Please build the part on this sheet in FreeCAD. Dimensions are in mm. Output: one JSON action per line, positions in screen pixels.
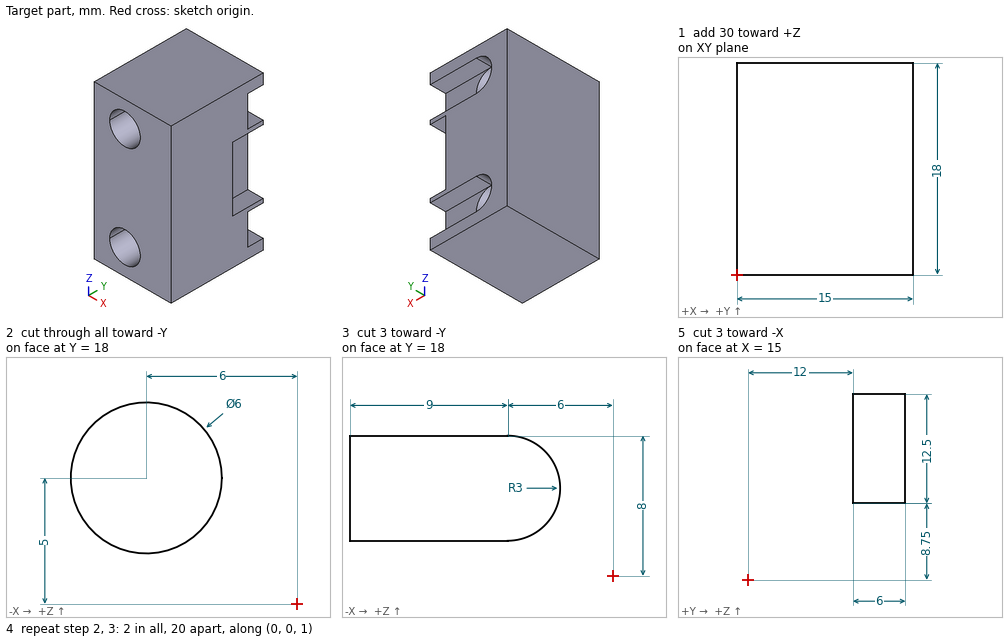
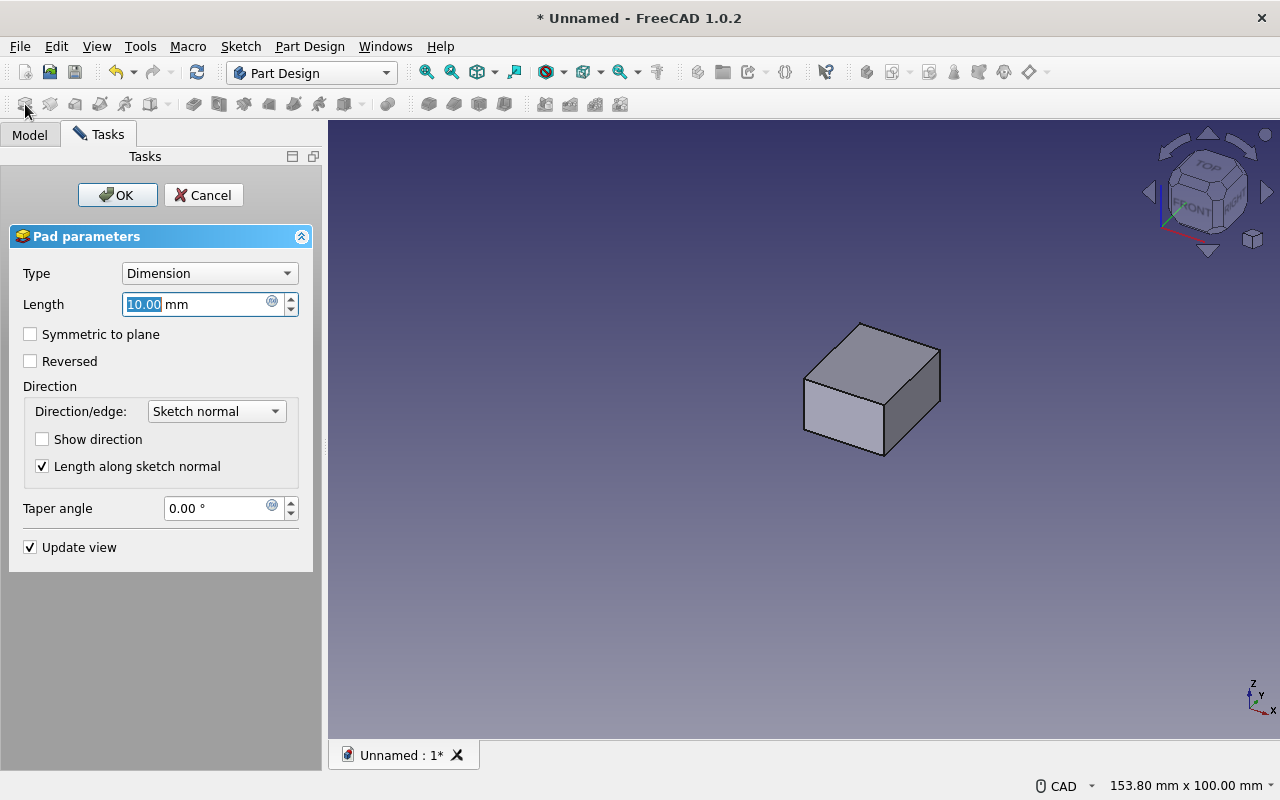
{"action": "type", "text": "30"}
{"action": "key", "text": "Tab"}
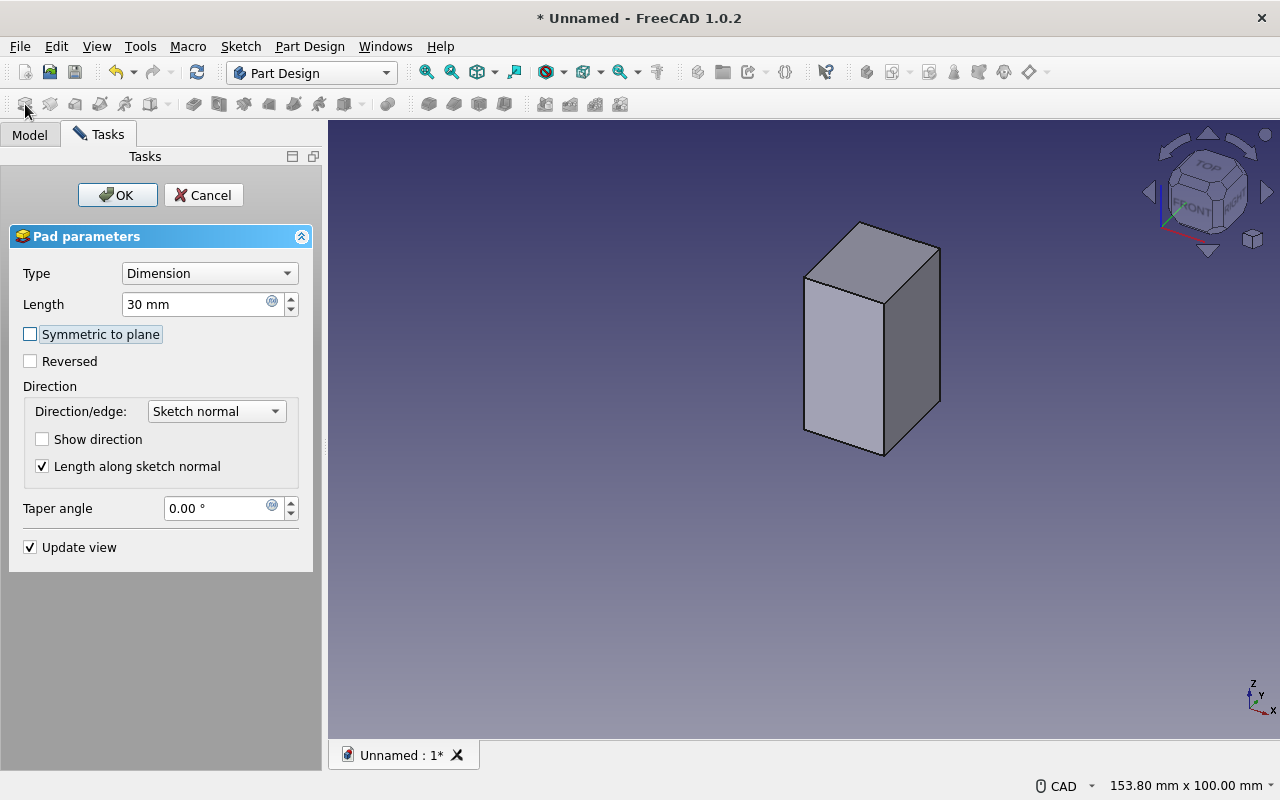
{"action": "left_click", "coordinate": [118, 195]}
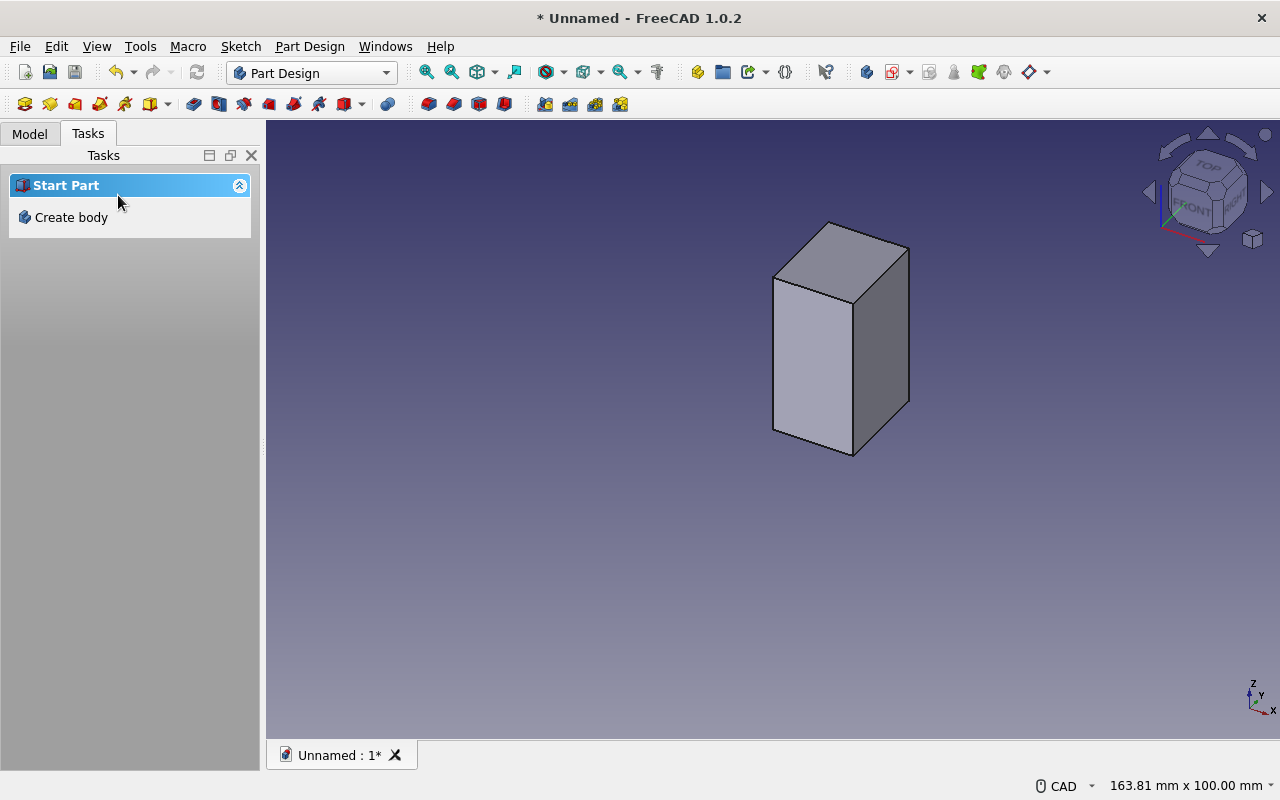
{"action": "left_click", "coordinate": [427, 72]}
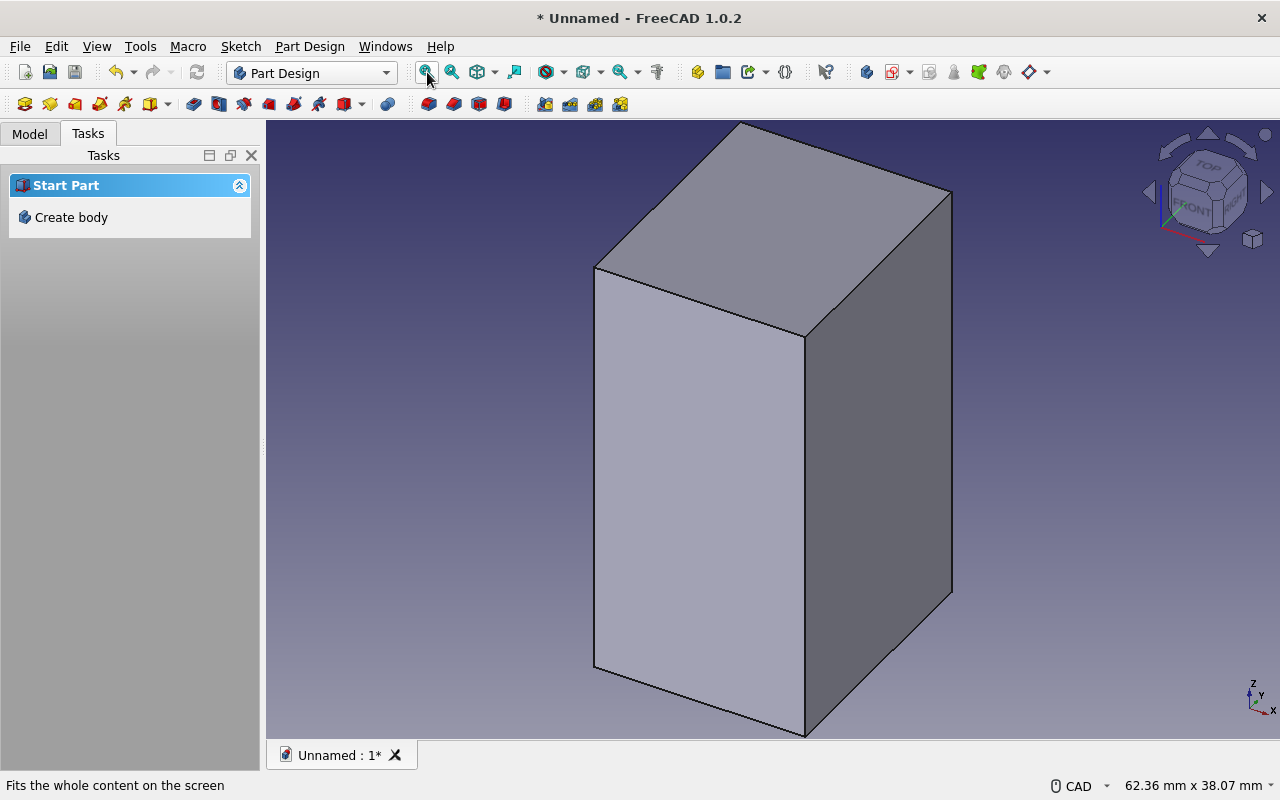
{"action": "key", "text": "4"}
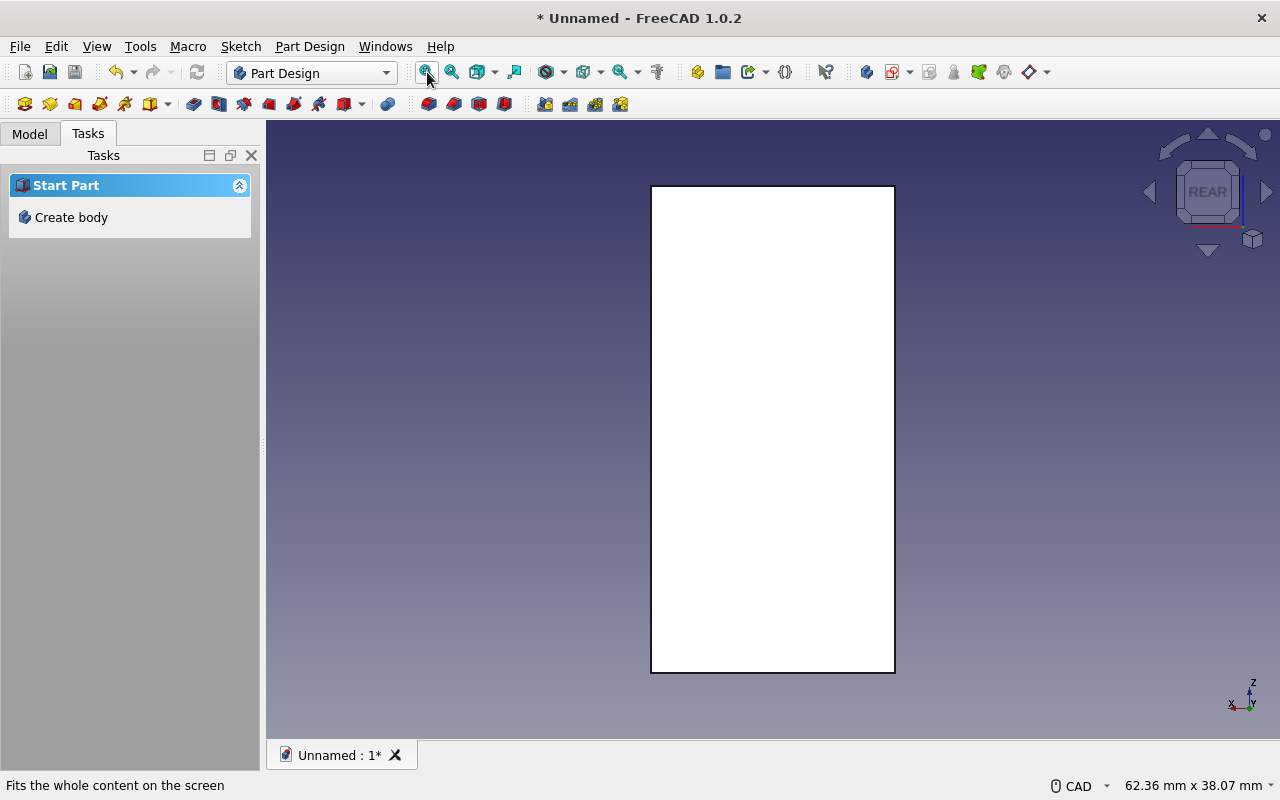
{"action": "left_click", "coordinate": [773, 359]}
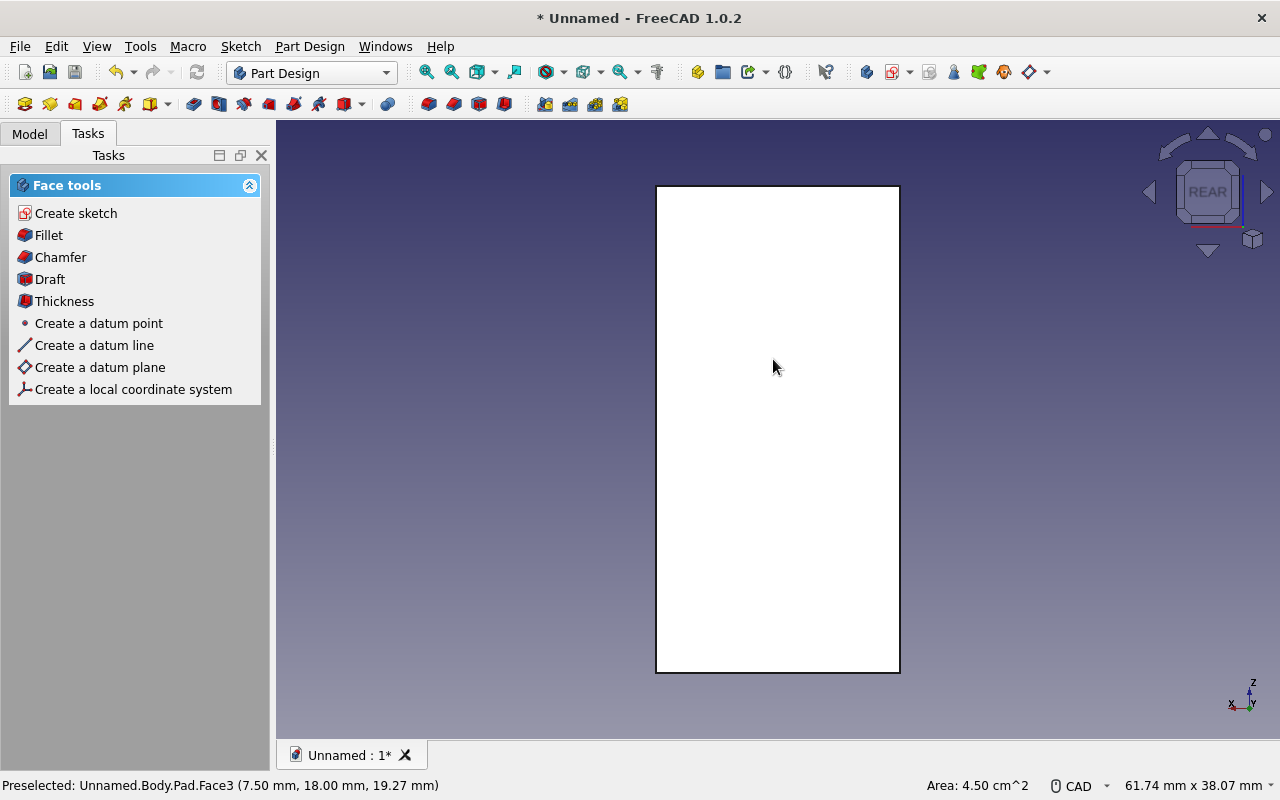
{"action": "left_click", "coordinate": [892, 72]}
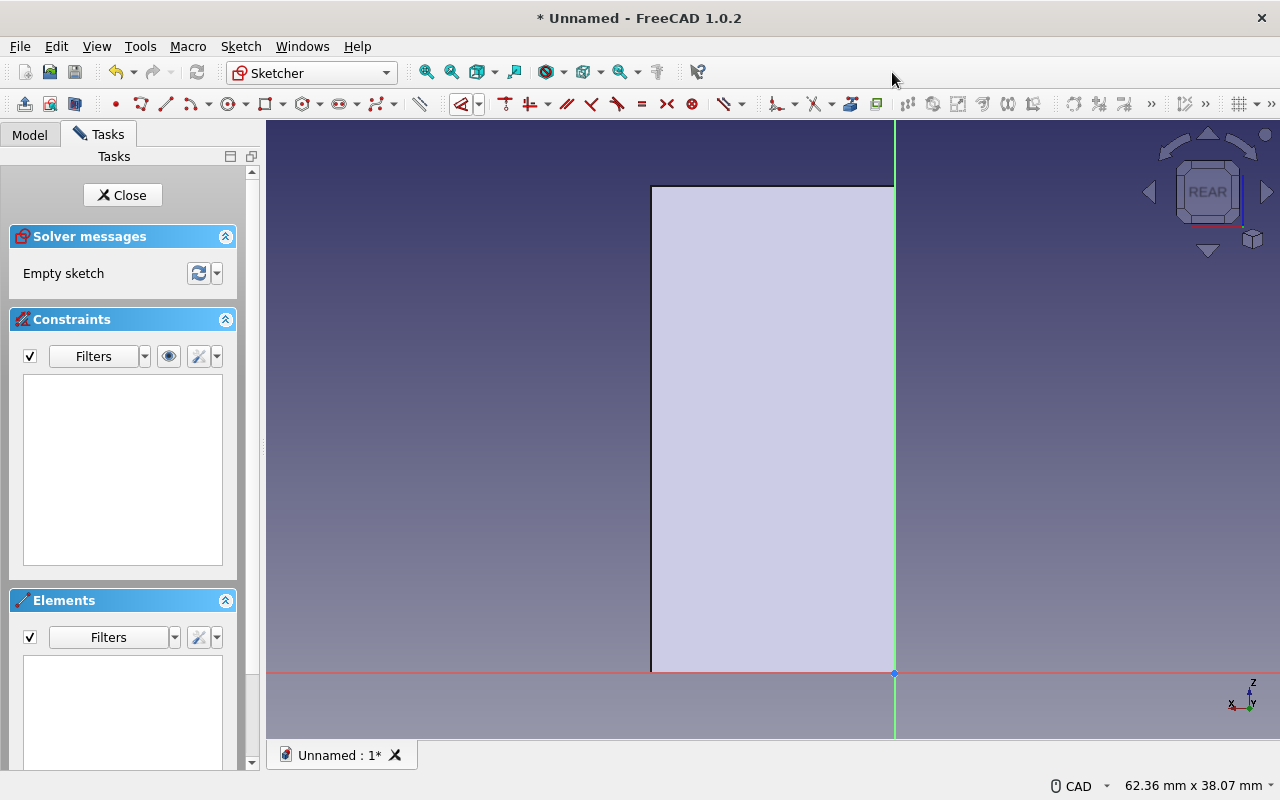
{"action": "scroll", "coordinate": [872, 685], "scroll_direction": "up", "scroll_amount": 6}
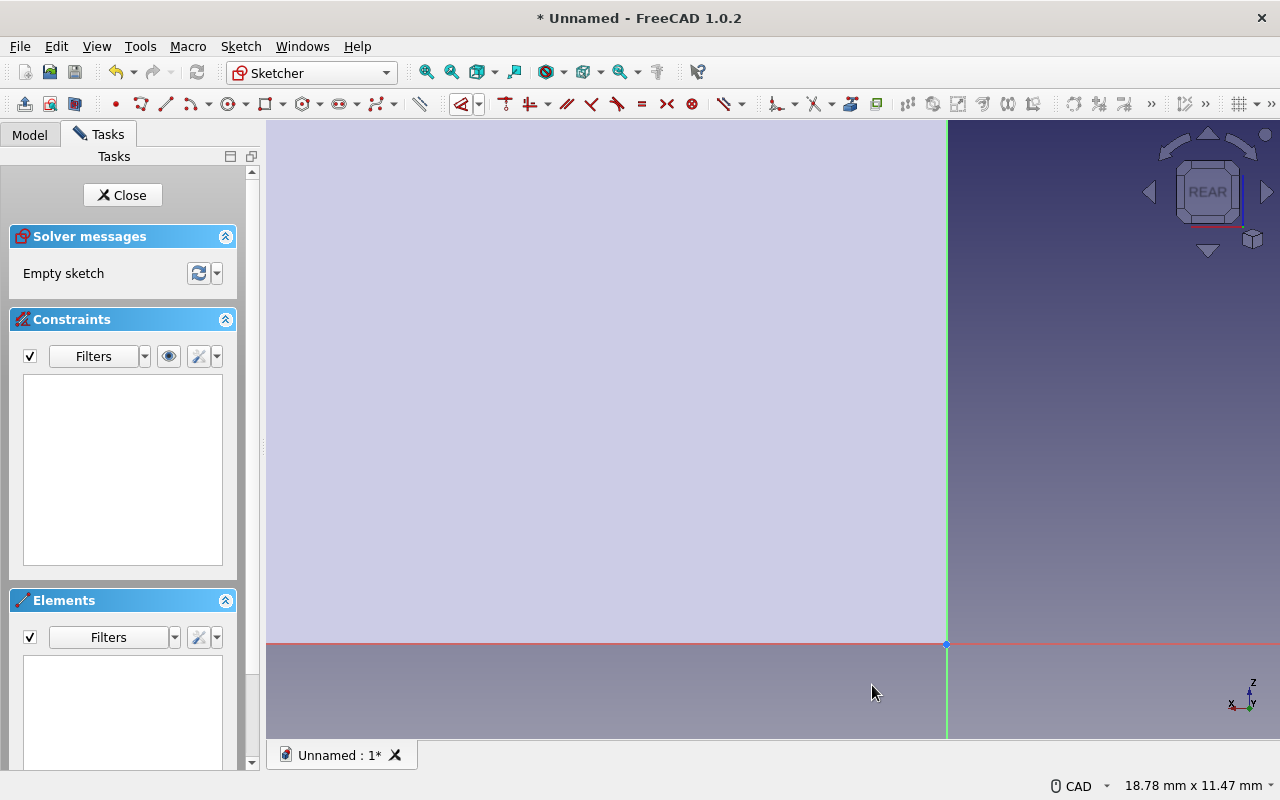
{"action": "left_click", "coordinate": [228, 104]}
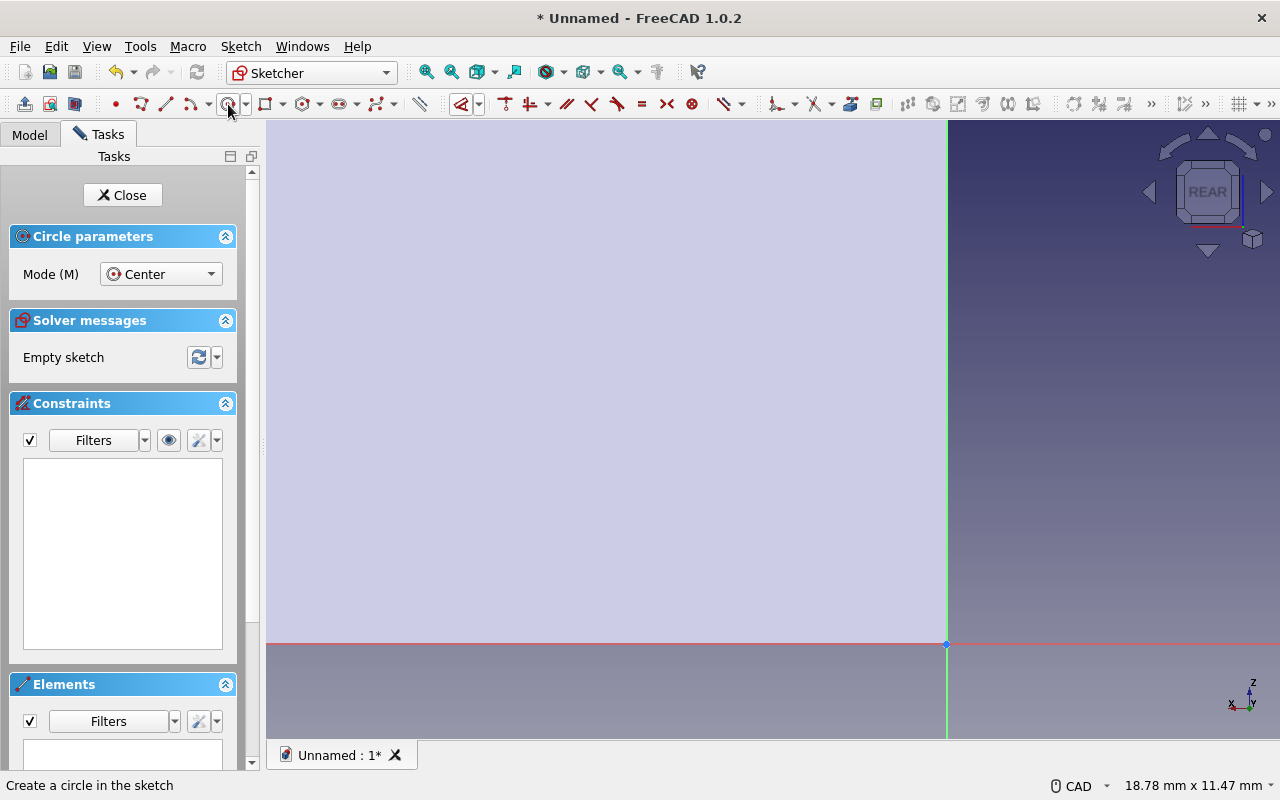
{"action": "left_click", "coordinate": [623, 374]}
{"action": "mouse_move", "coordinate": [737, 260]}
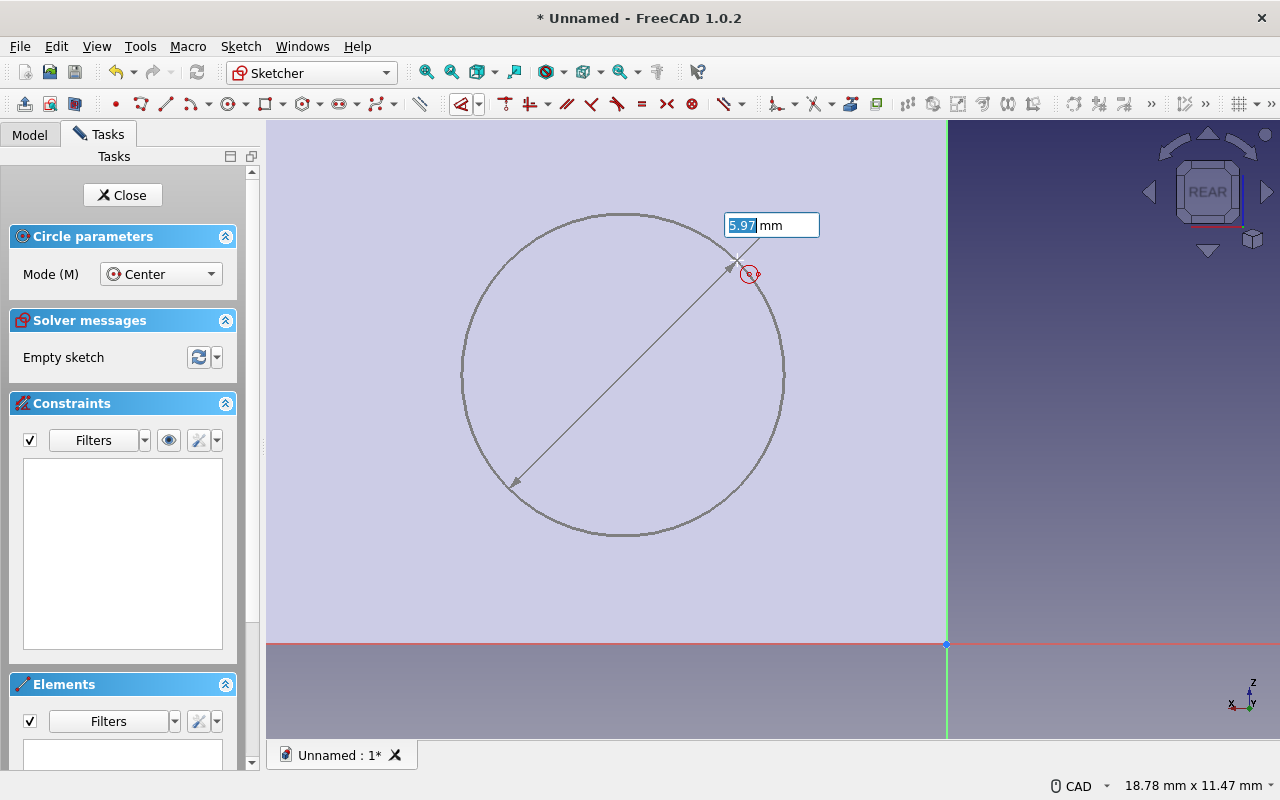
{"action": "type", "text": "6"}
{"action": "key", "text": "Return"}
{"action": "key", "text": "Escape"}